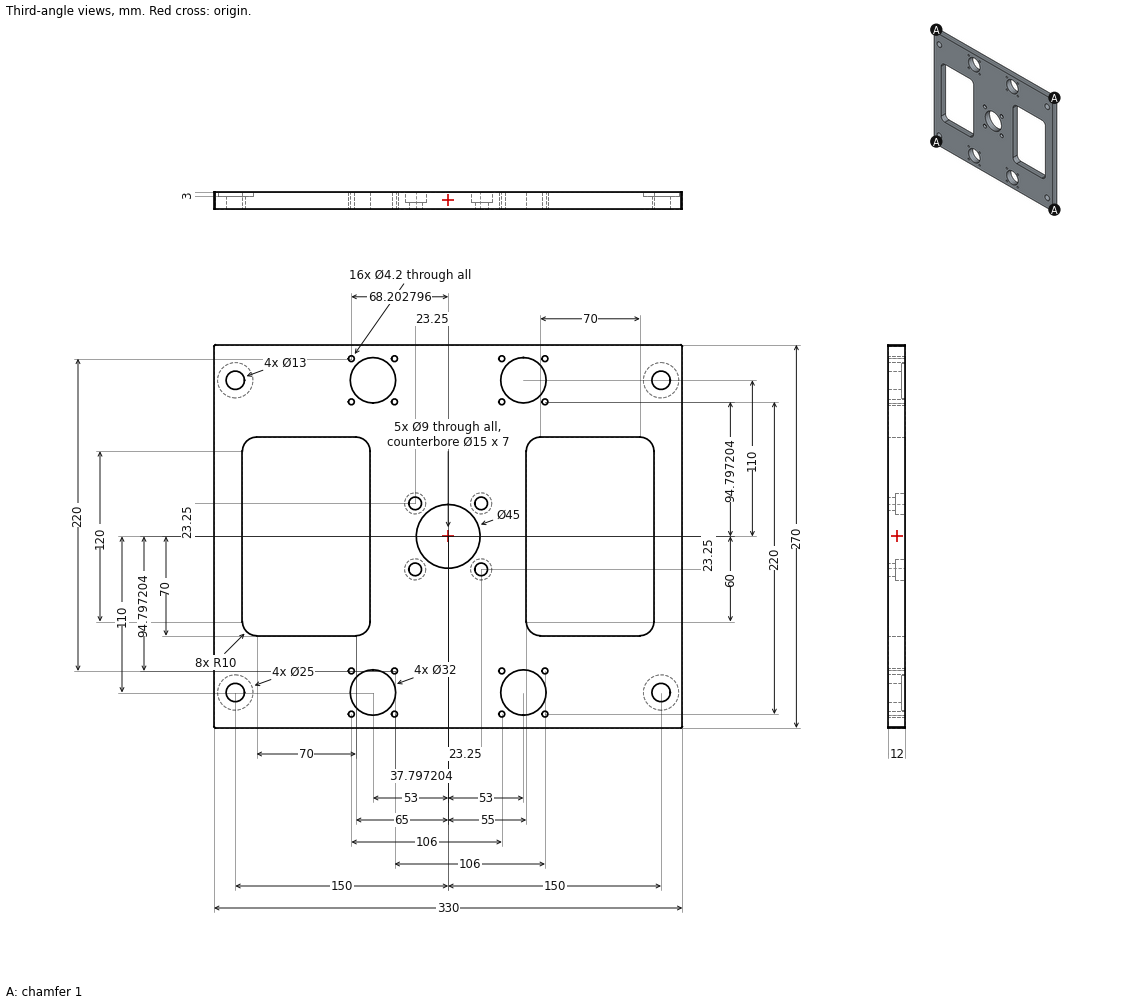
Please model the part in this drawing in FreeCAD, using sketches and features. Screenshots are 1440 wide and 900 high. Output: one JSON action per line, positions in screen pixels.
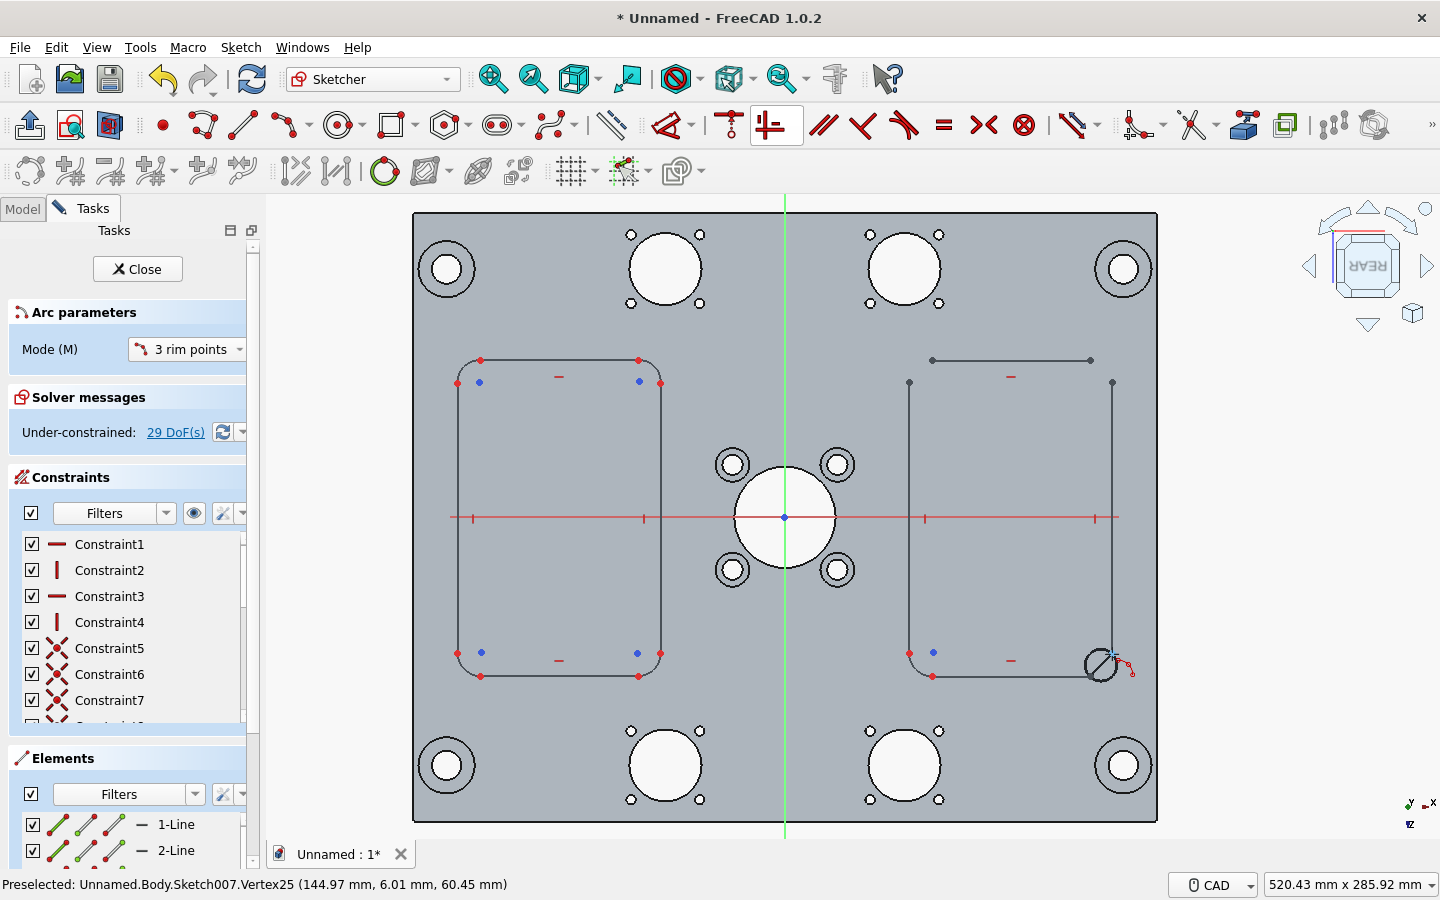
{"action": "scroll", "coordinate": [1105, 669], "scroll_direction": "up", "scroll_amount": 5}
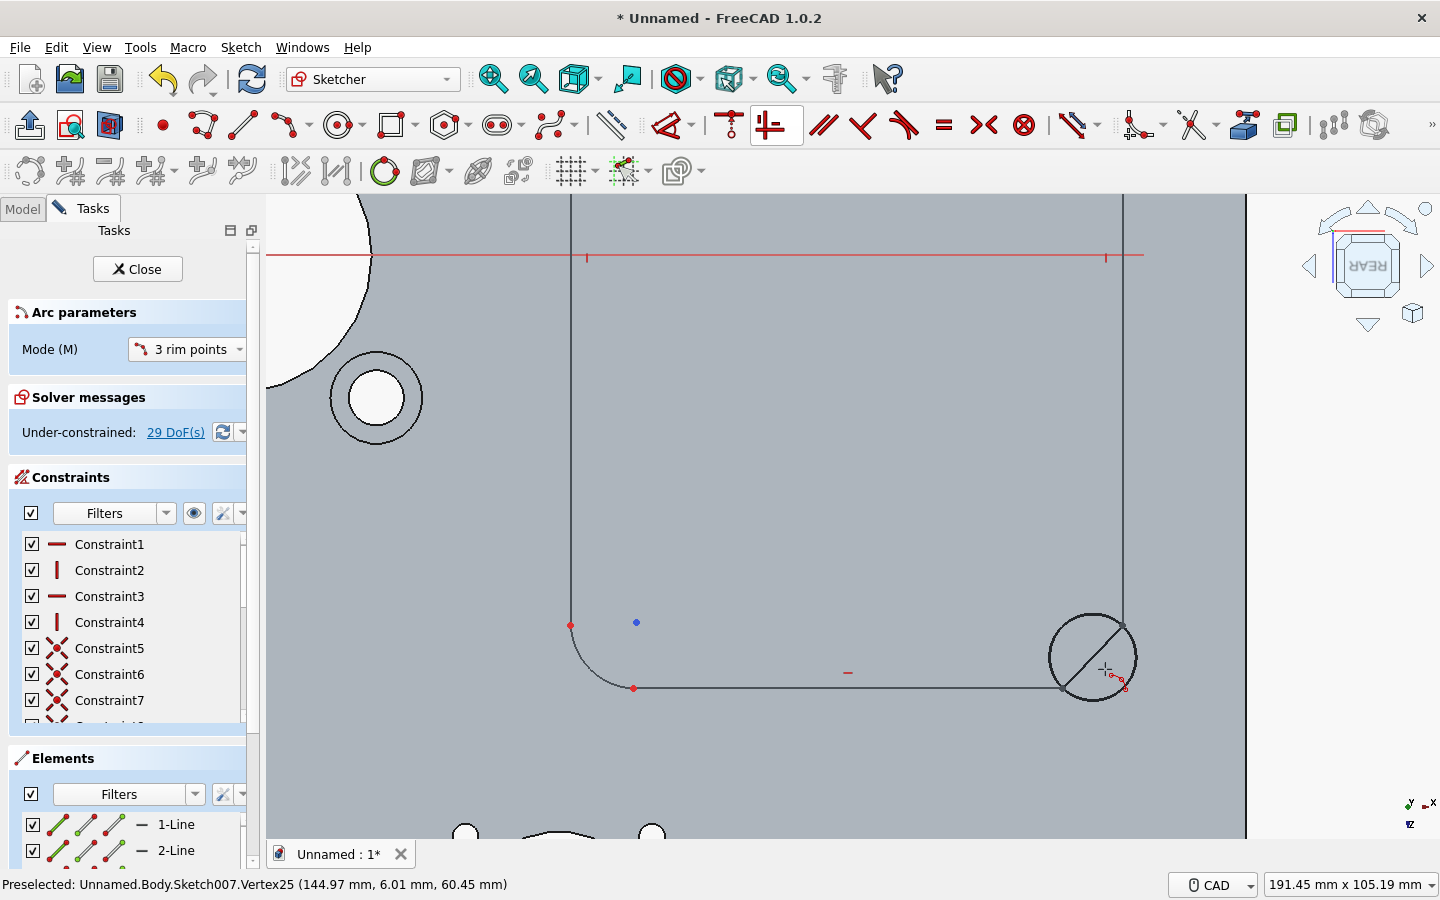
{"action": "left_click", "coordinate": [1105, 667]}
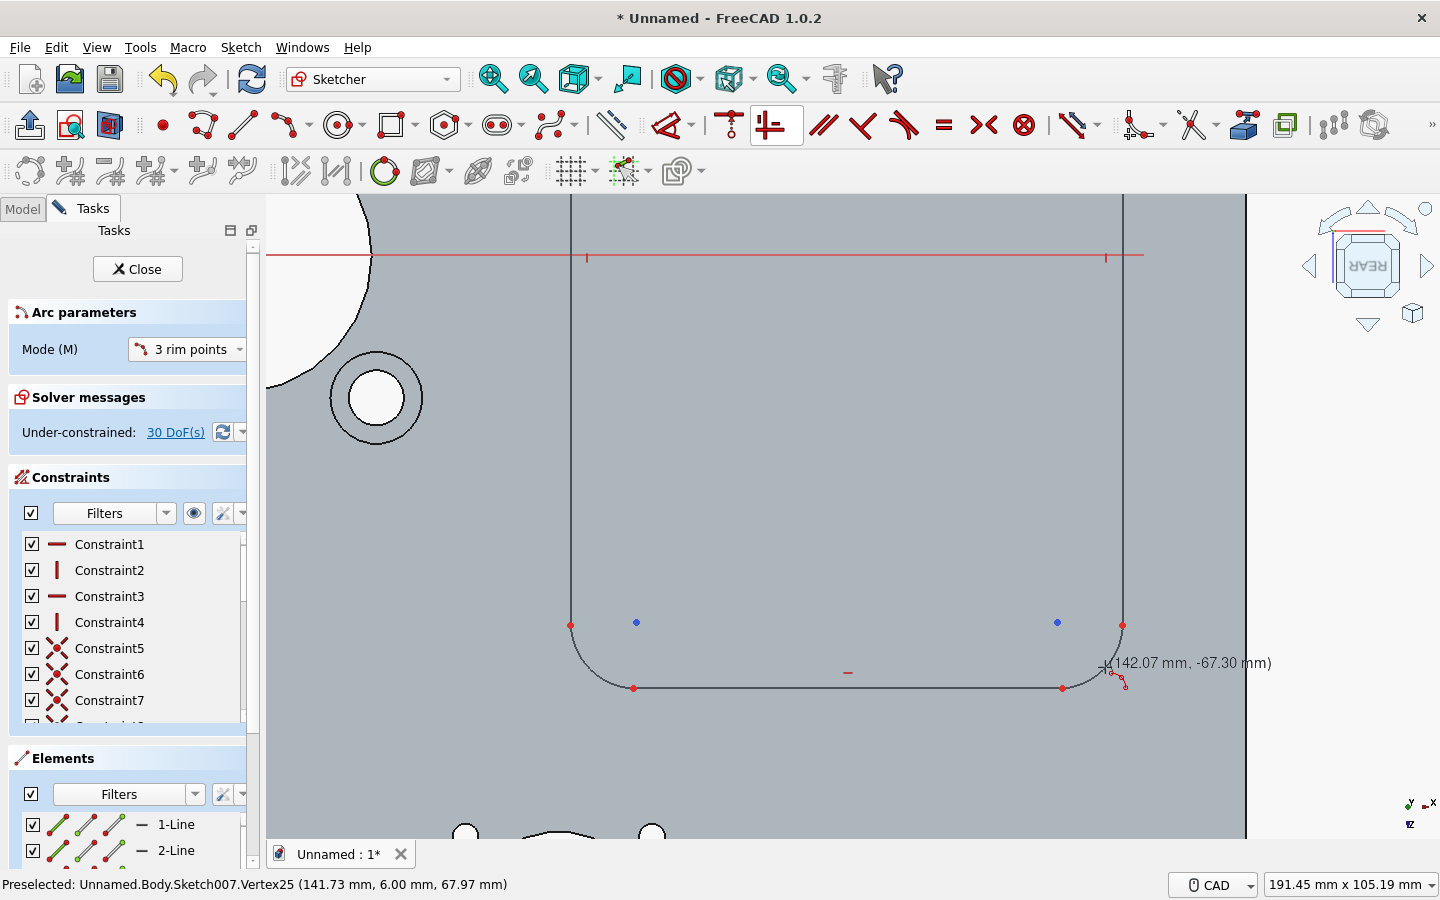
{"action": "scroll", "coordinate": [1105, 669], "scroll_direction": "down", "scroll_amount": 5}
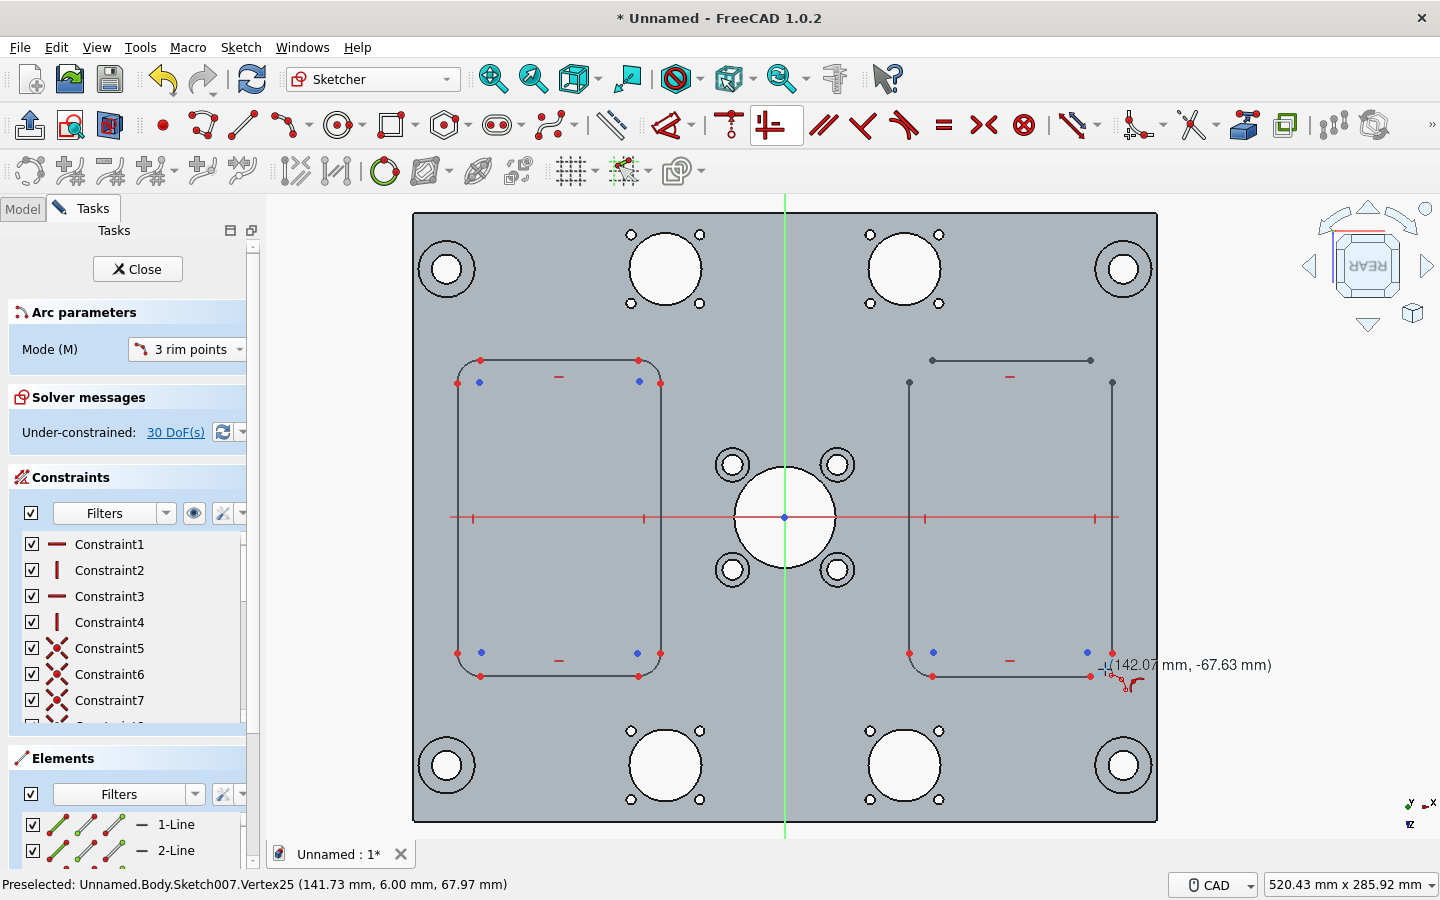
{"action": "left_click", "coordinate": [1112, 383]}
{"action": "left_click", "coordinate": [1090, 361]}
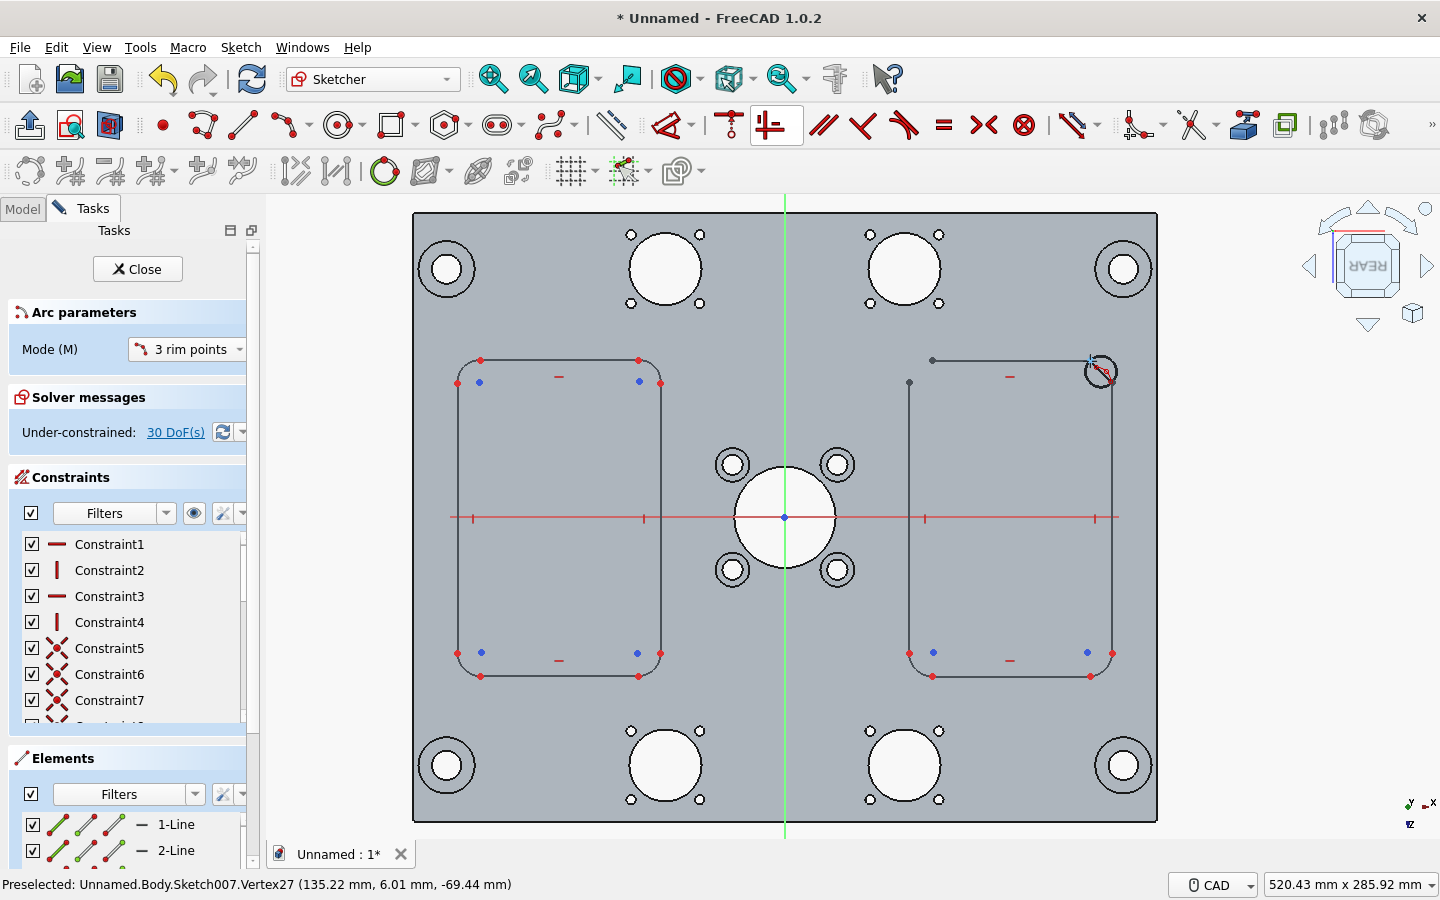
{"action": "scroll", "coordinate": [1105, 366], "scroll_direction": "up", "scroll_amount": 5}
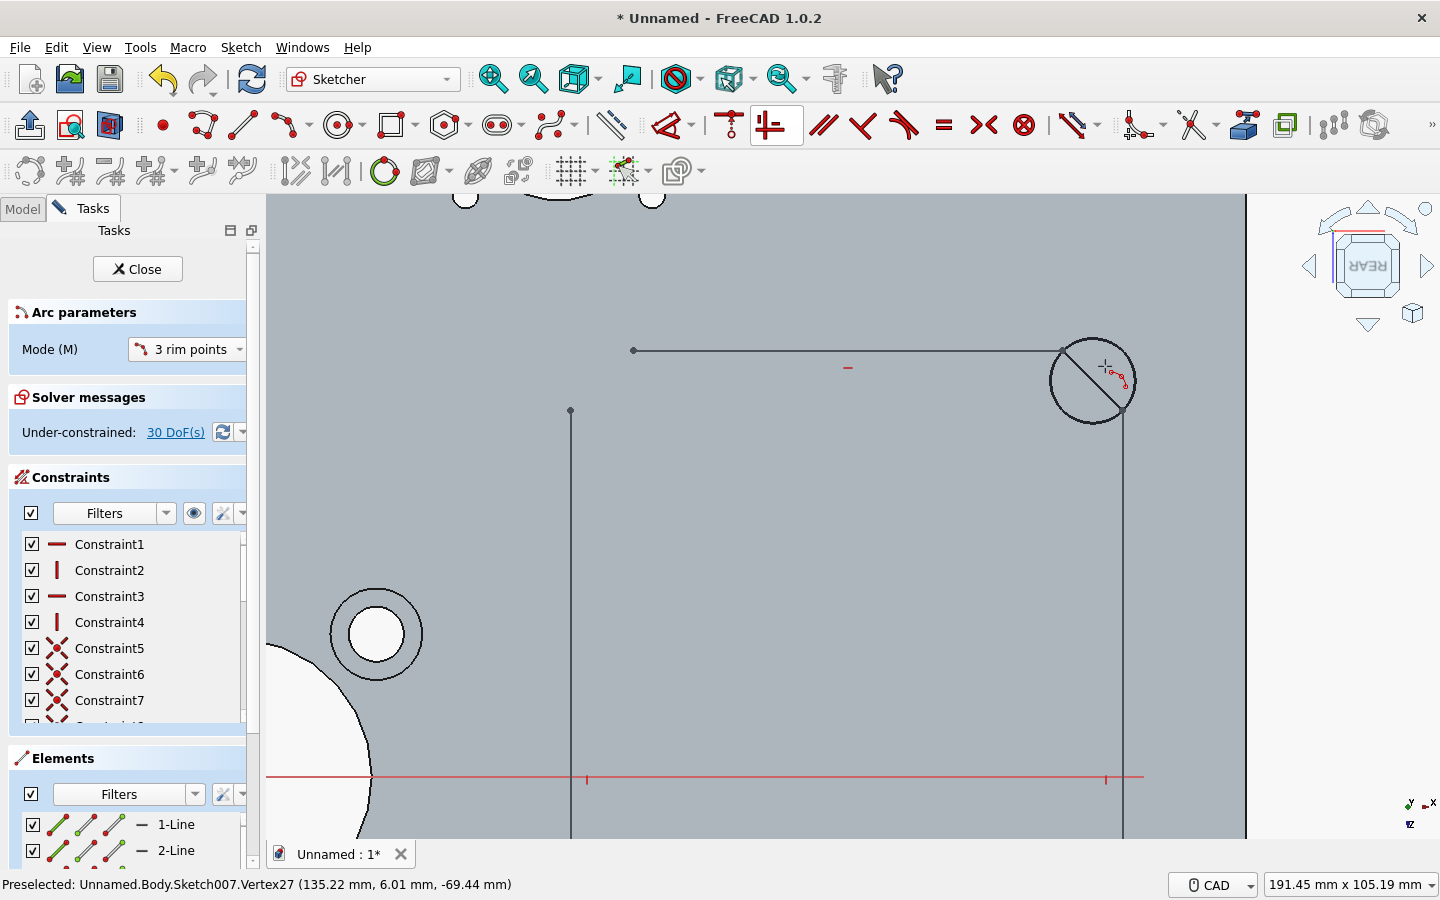
{"action": "left_click", "coordinate": [1105, 365]}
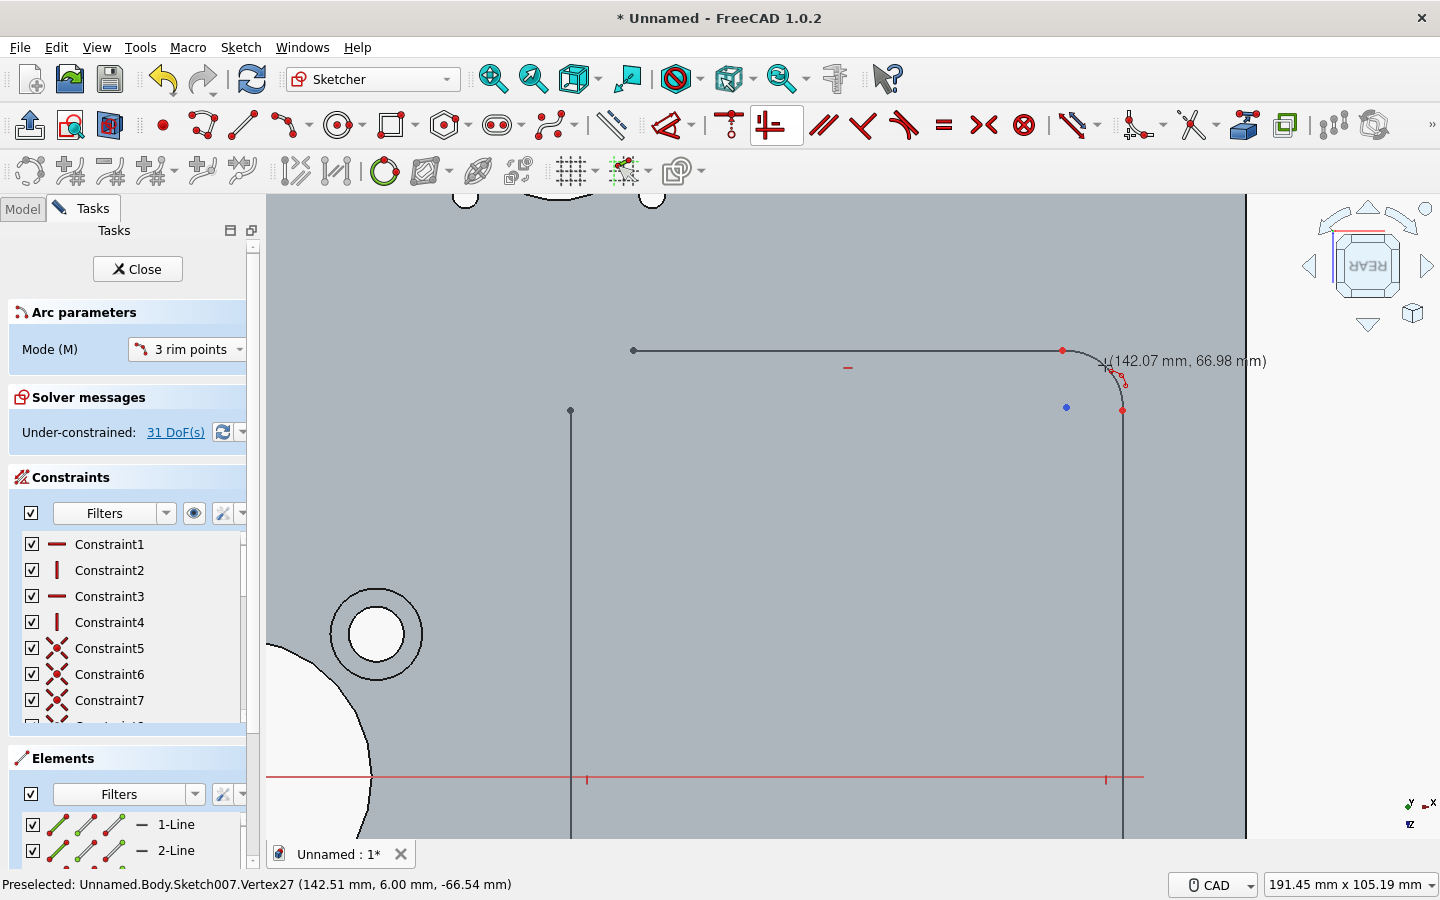
{"action": "left_click", "coordinate": [634, 351]}
{"action": "left_click", "coordinate": [571, 411]}
{"action": "left_click", "coordinate": [589, 365]}
{"action": "key", "text": "Escape"}